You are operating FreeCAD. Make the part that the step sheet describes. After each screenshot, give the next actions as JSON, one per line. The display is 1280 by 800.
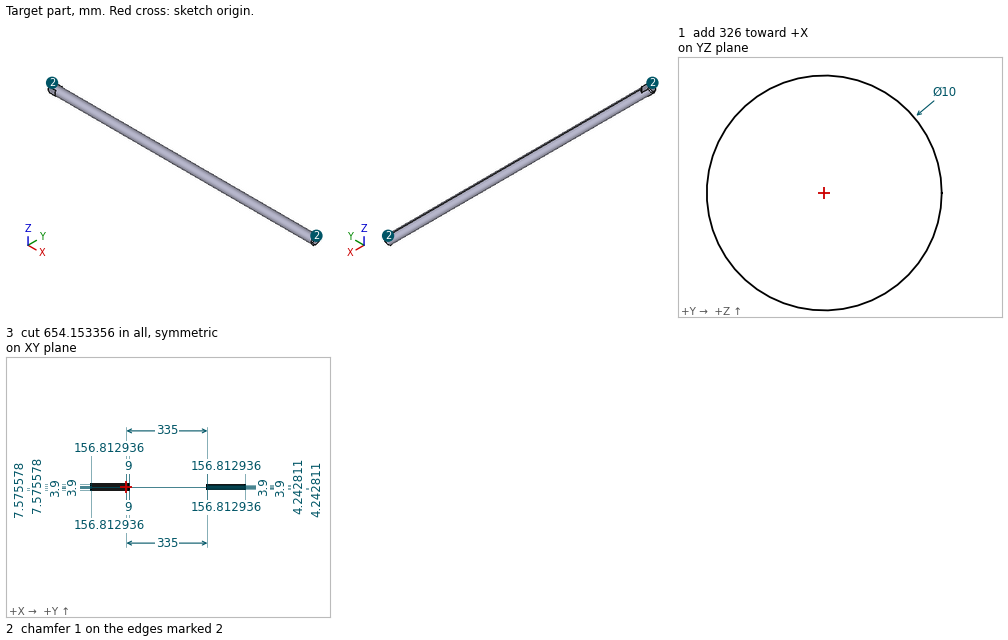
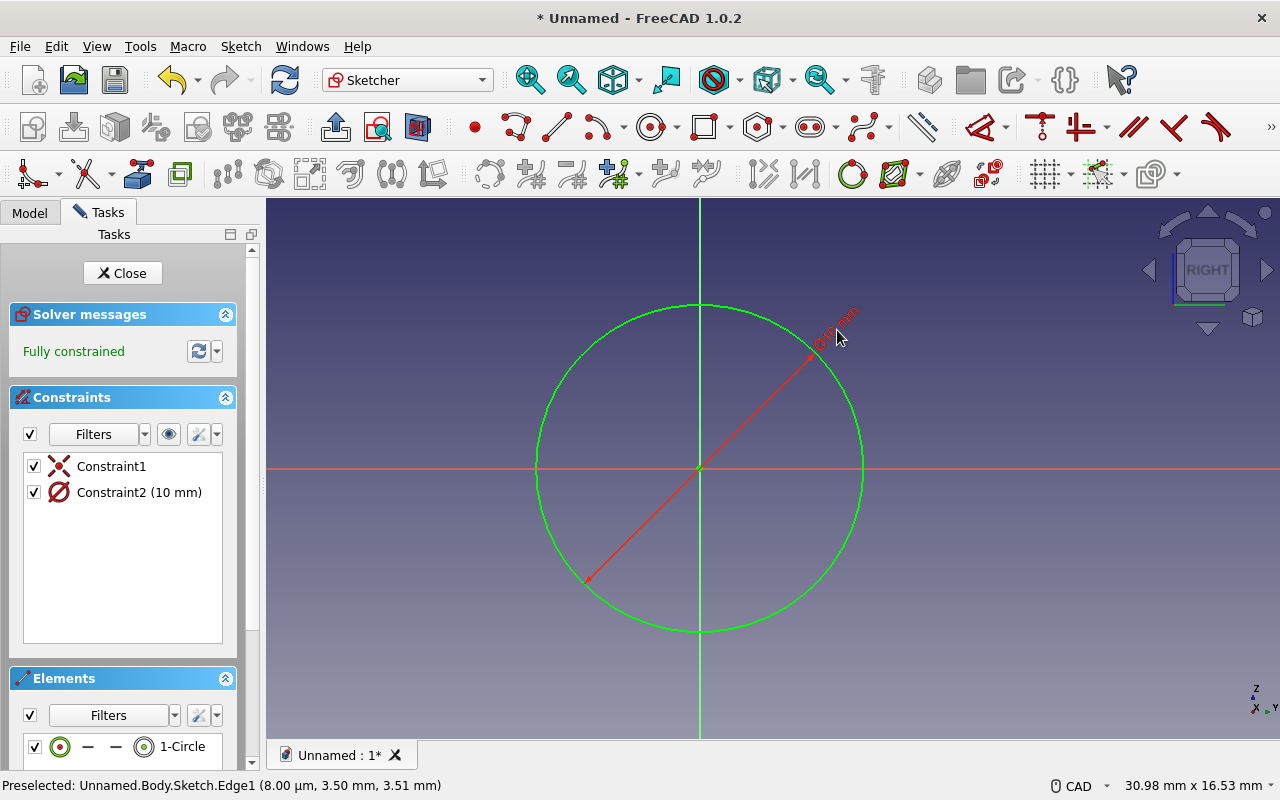
{"action": "left_click", "coordinate": [123, 273]}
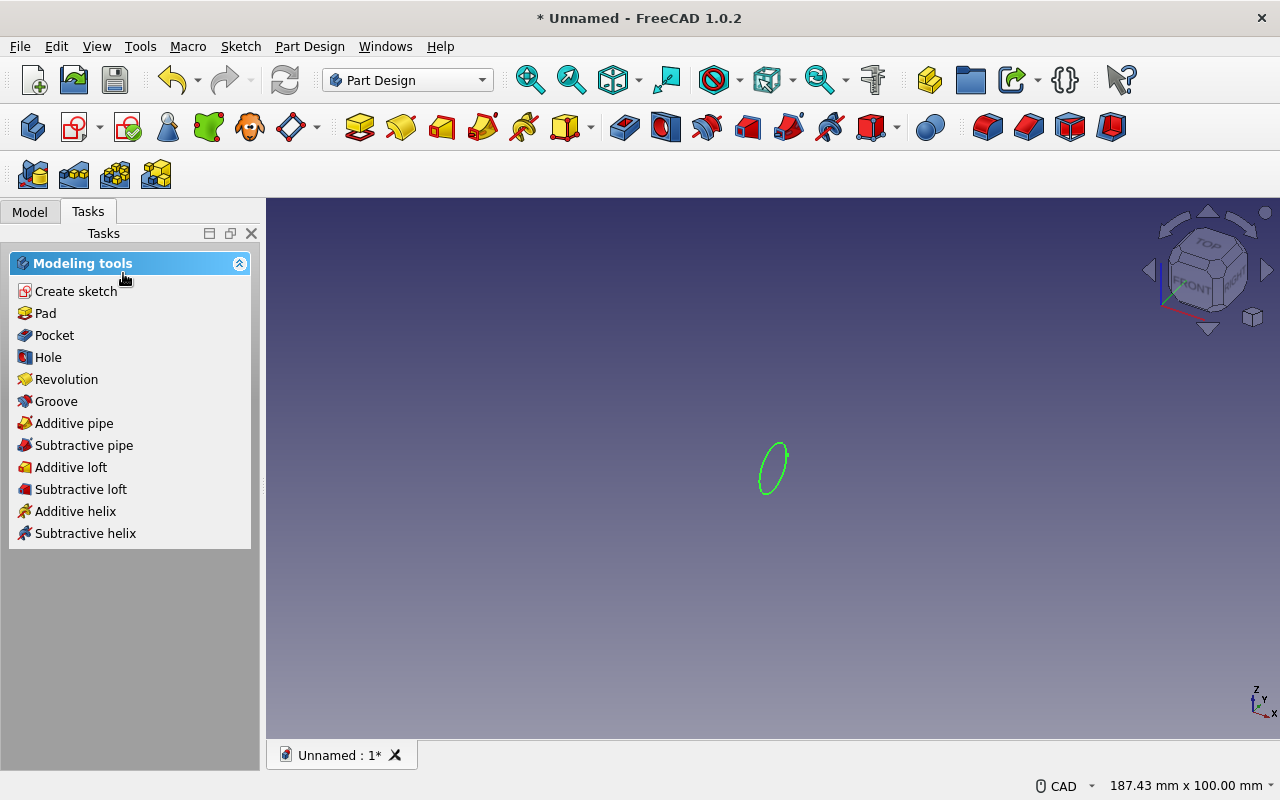
{"action": "left_click", "coordinate": [360, 128]}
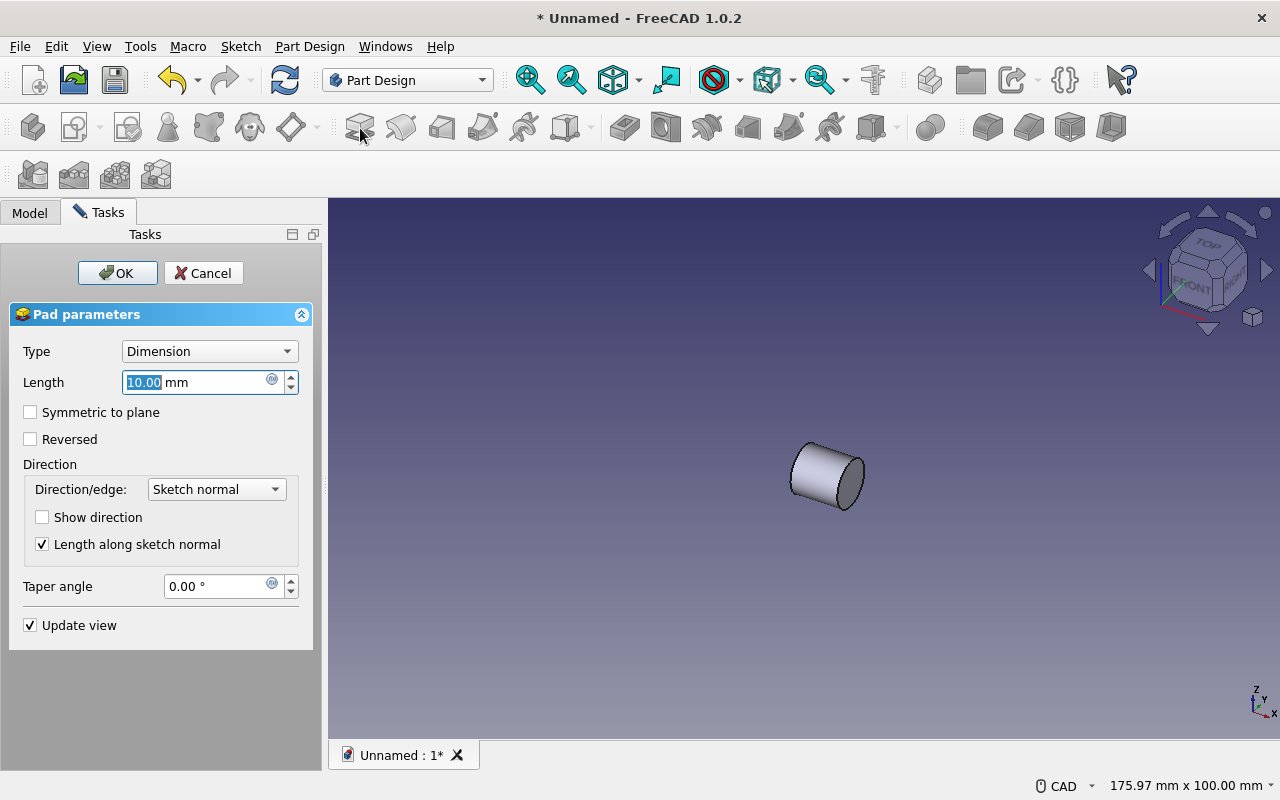
{"action": "type", "text": "326"}
{"action": "key", "text": "Tab"}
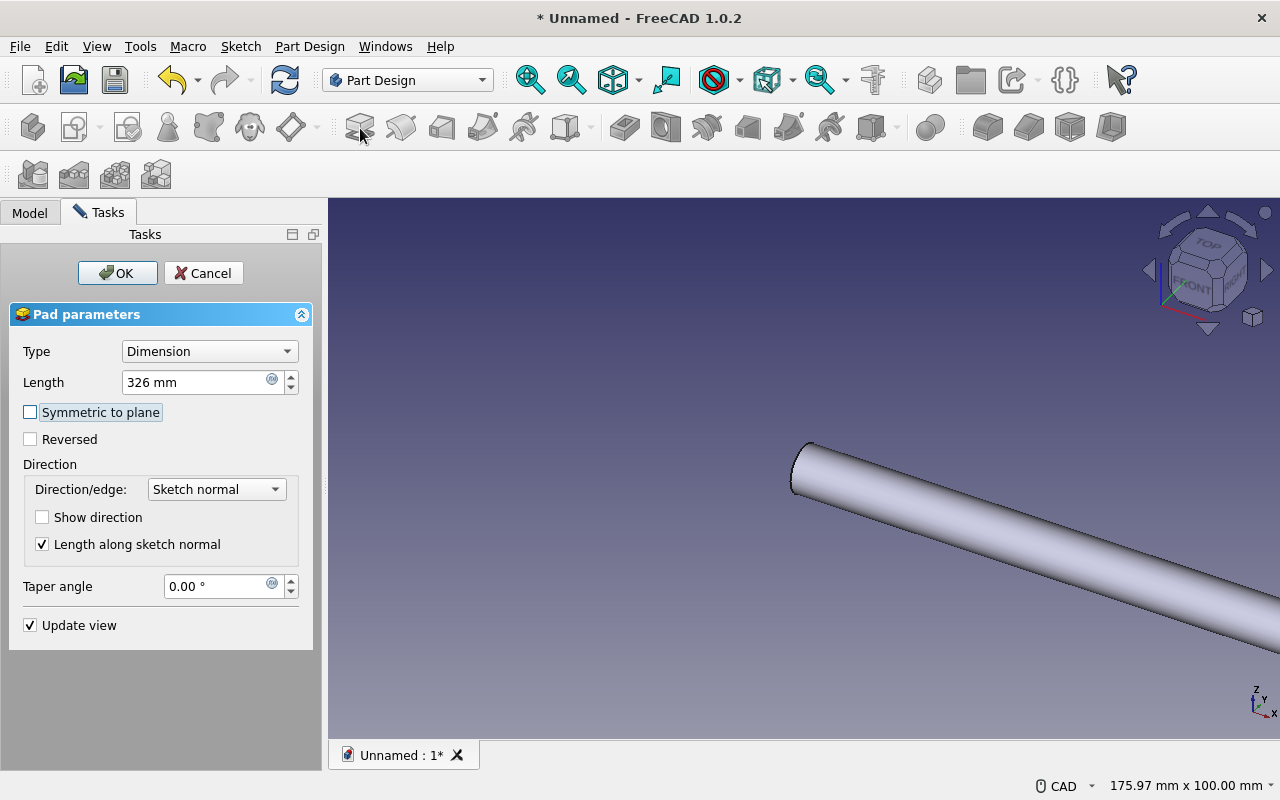
{"action": "left_click", "coordinate": [118, 273]}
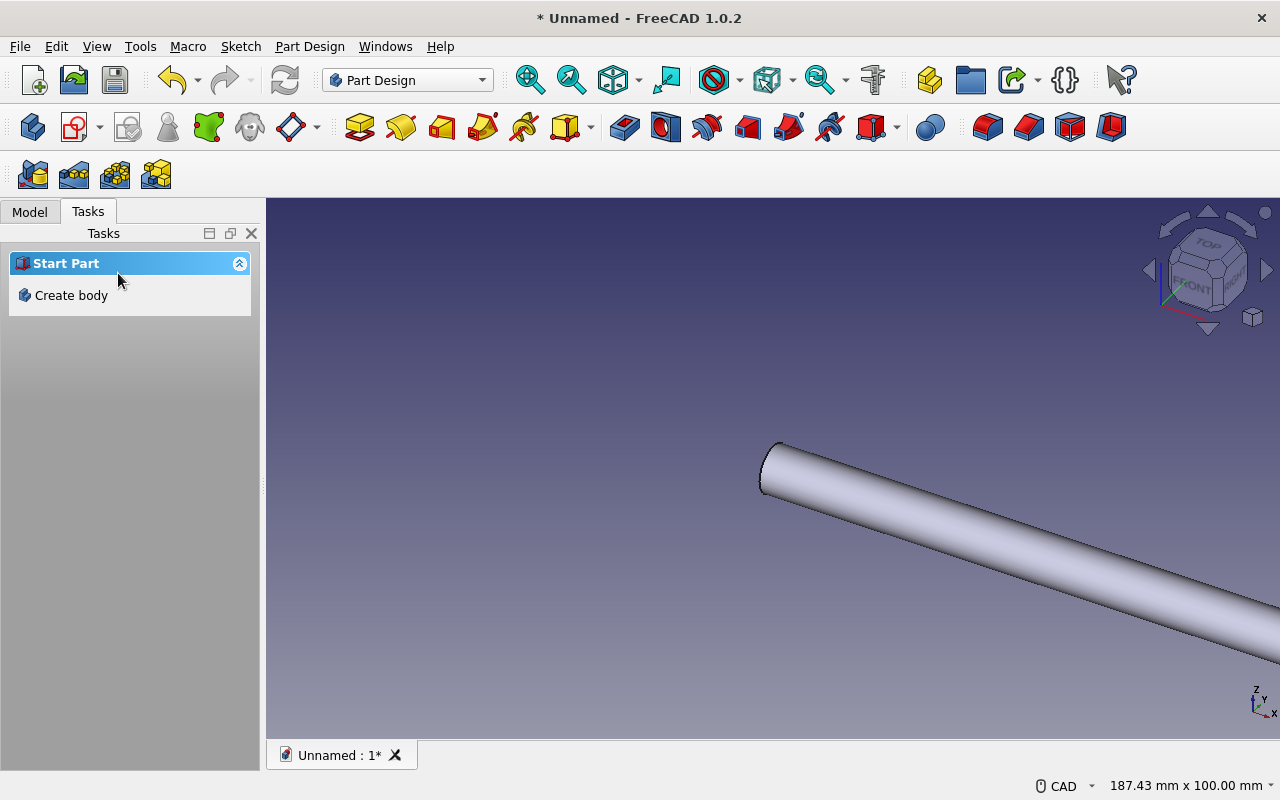
{"action": "key", "text": "v f"}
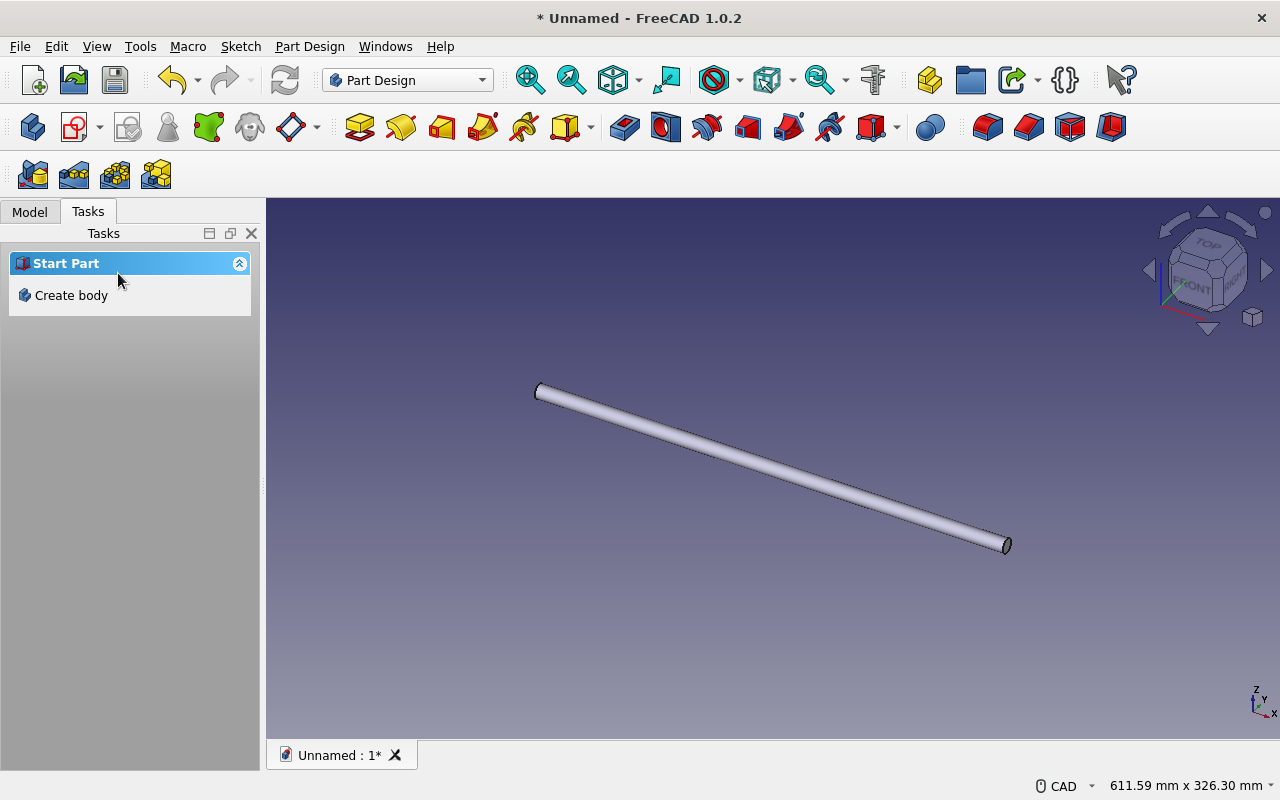
{"action": "left_click", "coordinate": [535, 394]}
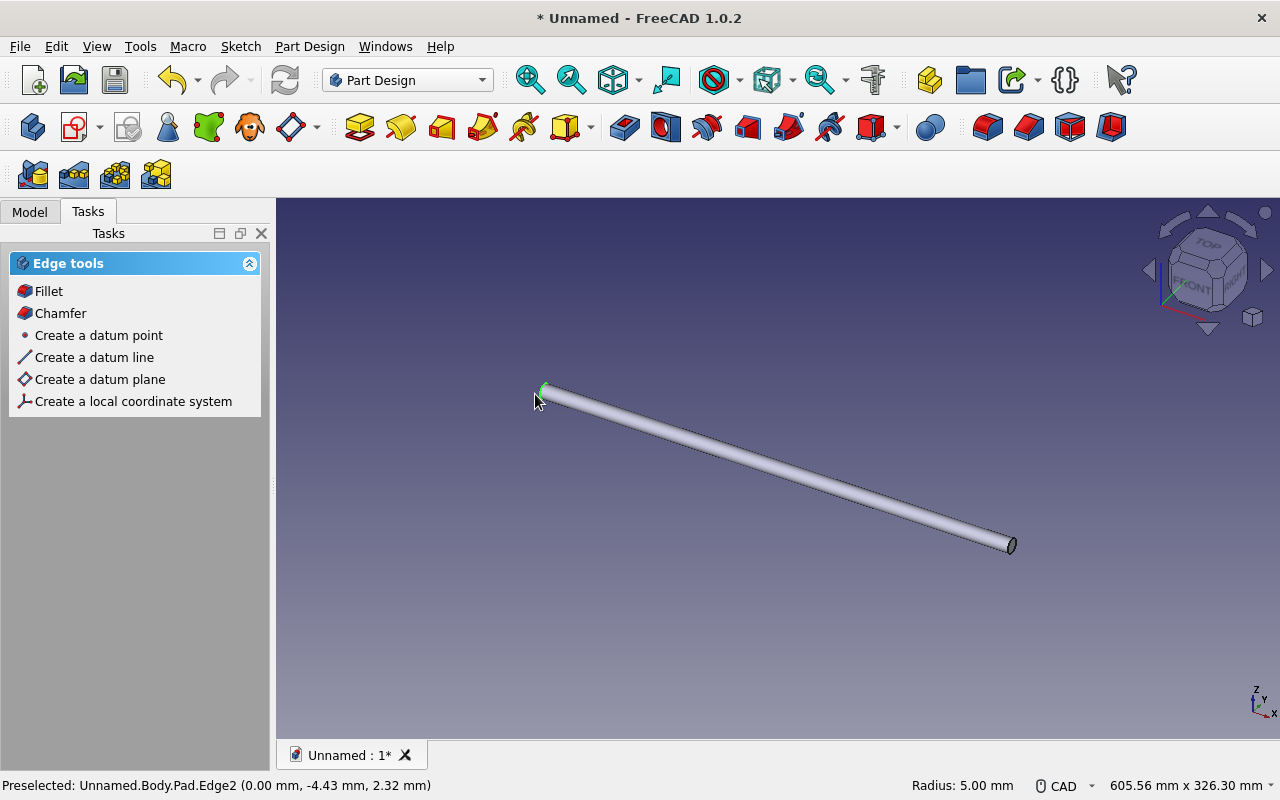
{"action": "left_click", "coordinate": [1008, 549], "text": "ctrl"}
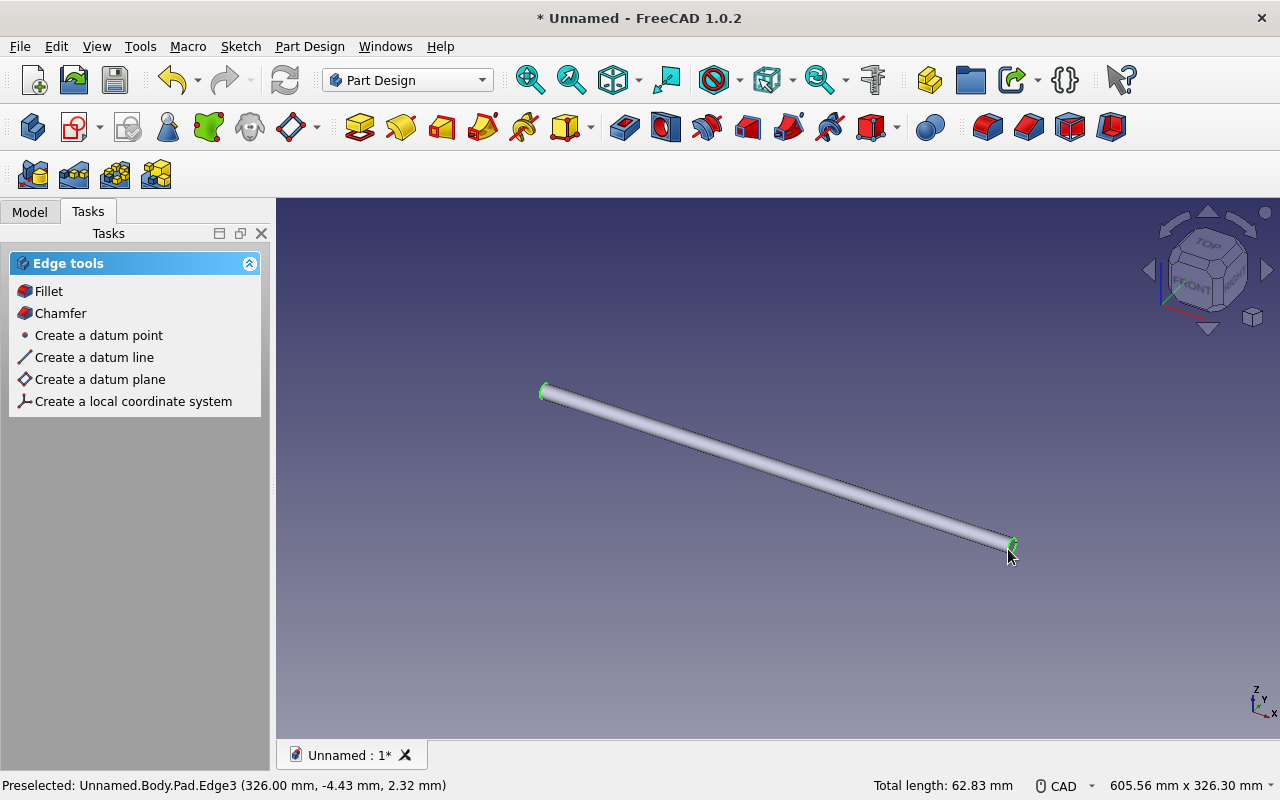
{"action": "left_click", "coordinate": [1029, 128]}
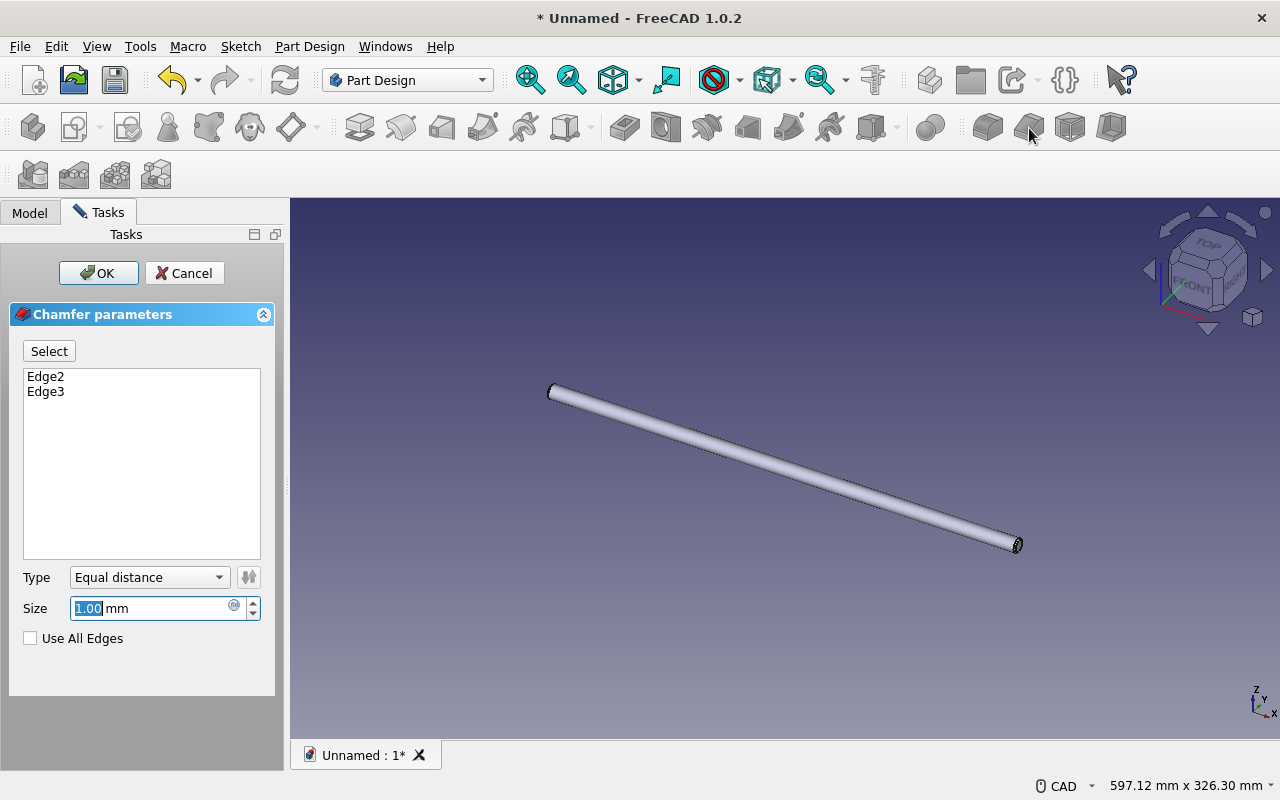
{"action": "type", "text": "1"}
{"action": "key", "text": "Tab"}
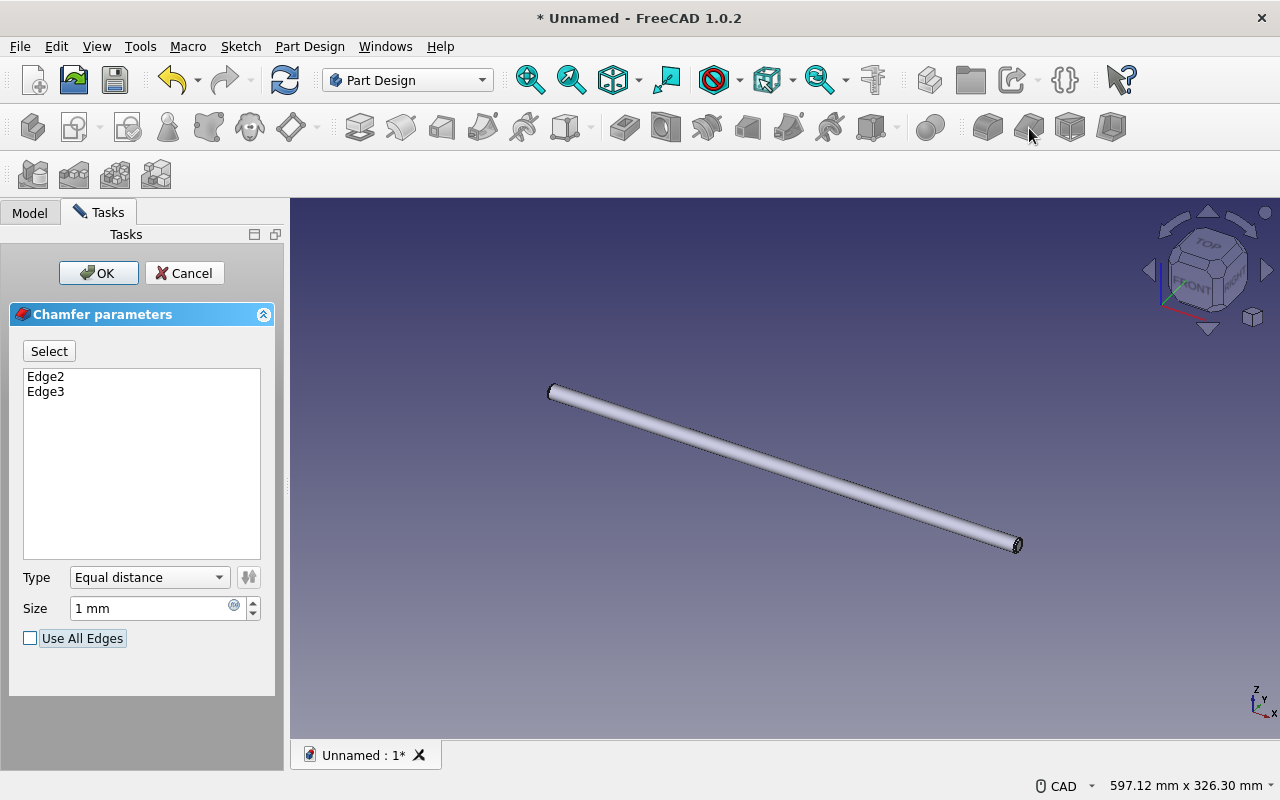
{"action": "left_click", "coordinate": [99, 273]}